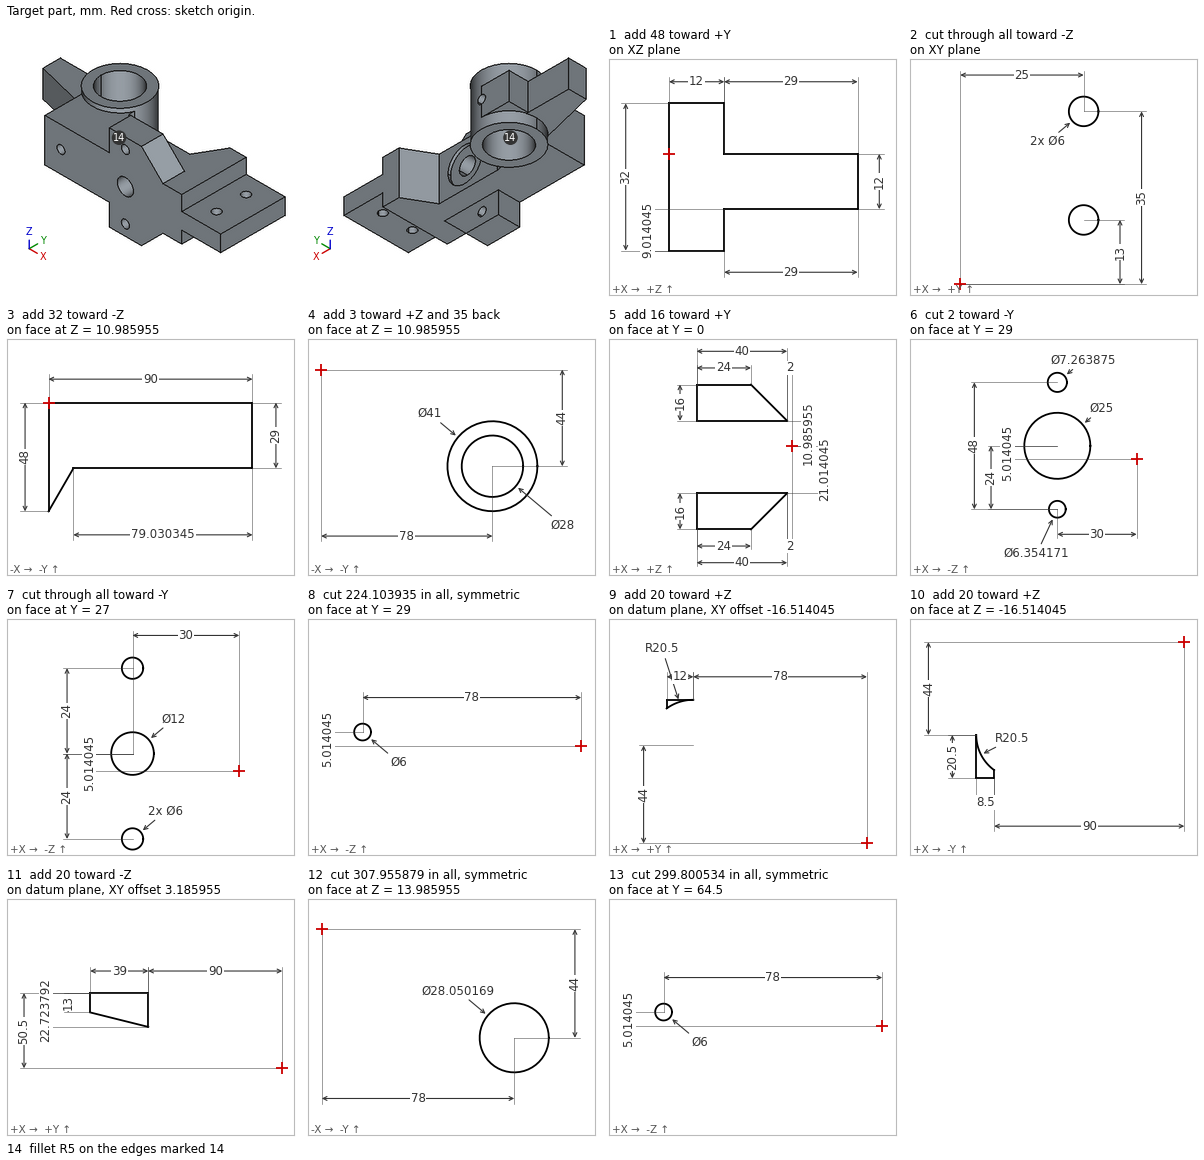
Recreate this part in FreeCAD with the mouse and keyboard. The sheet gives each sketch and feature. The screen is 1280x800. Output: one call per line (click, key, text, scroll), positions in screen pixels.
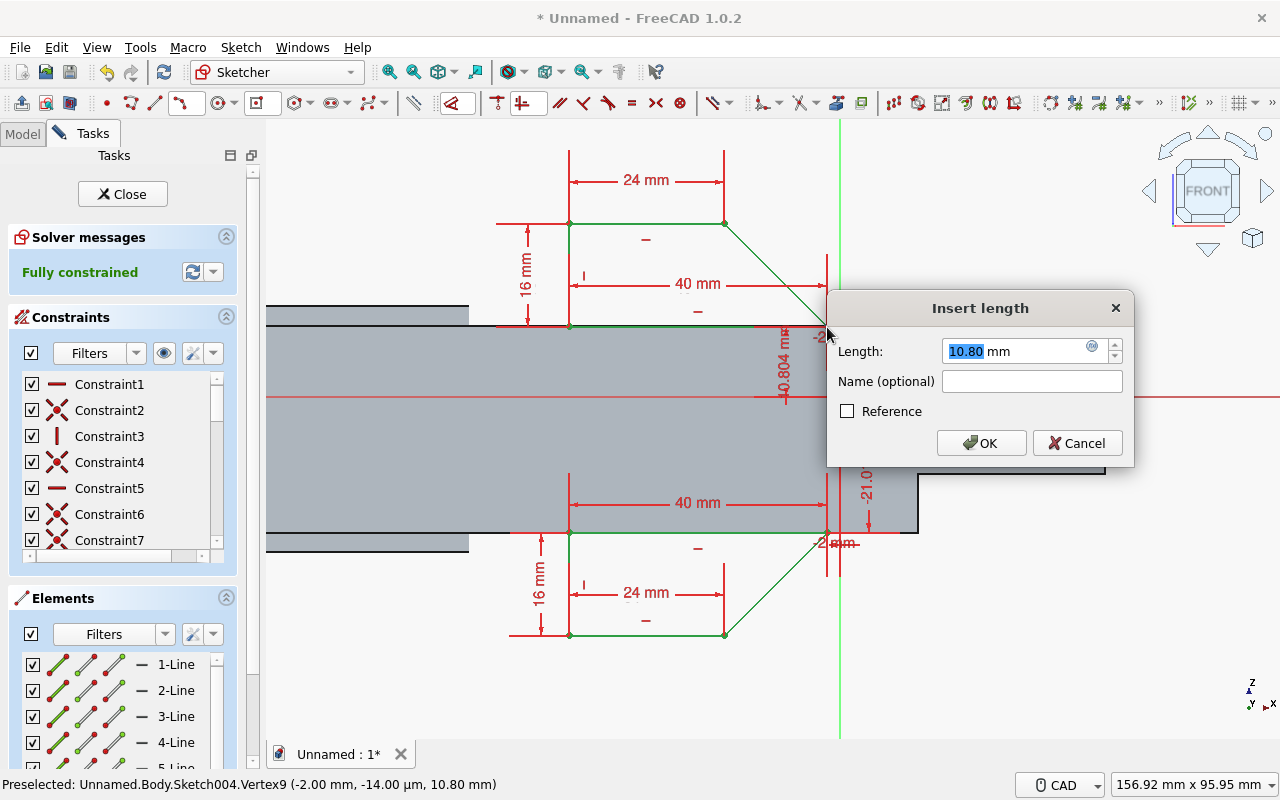
text(10.985955)
key(Return)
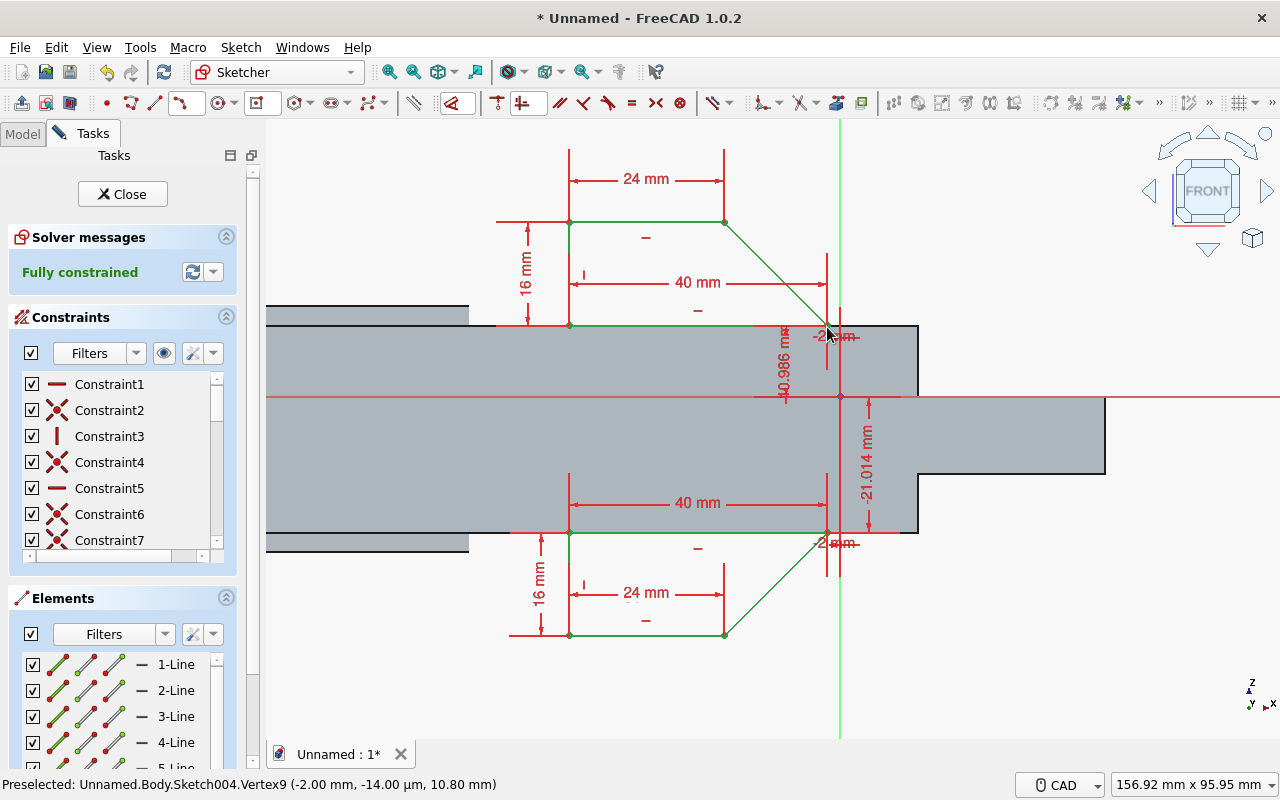
click(123, 194)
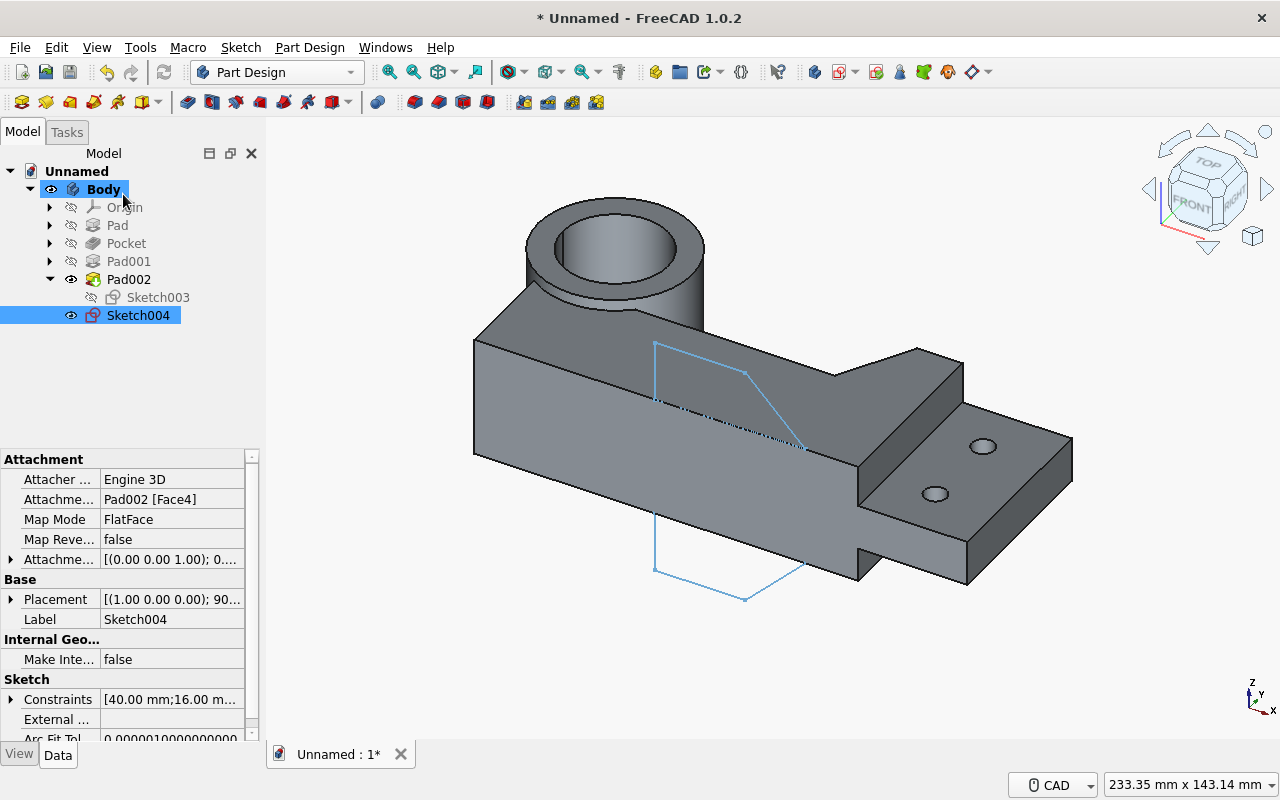
click(22, 102)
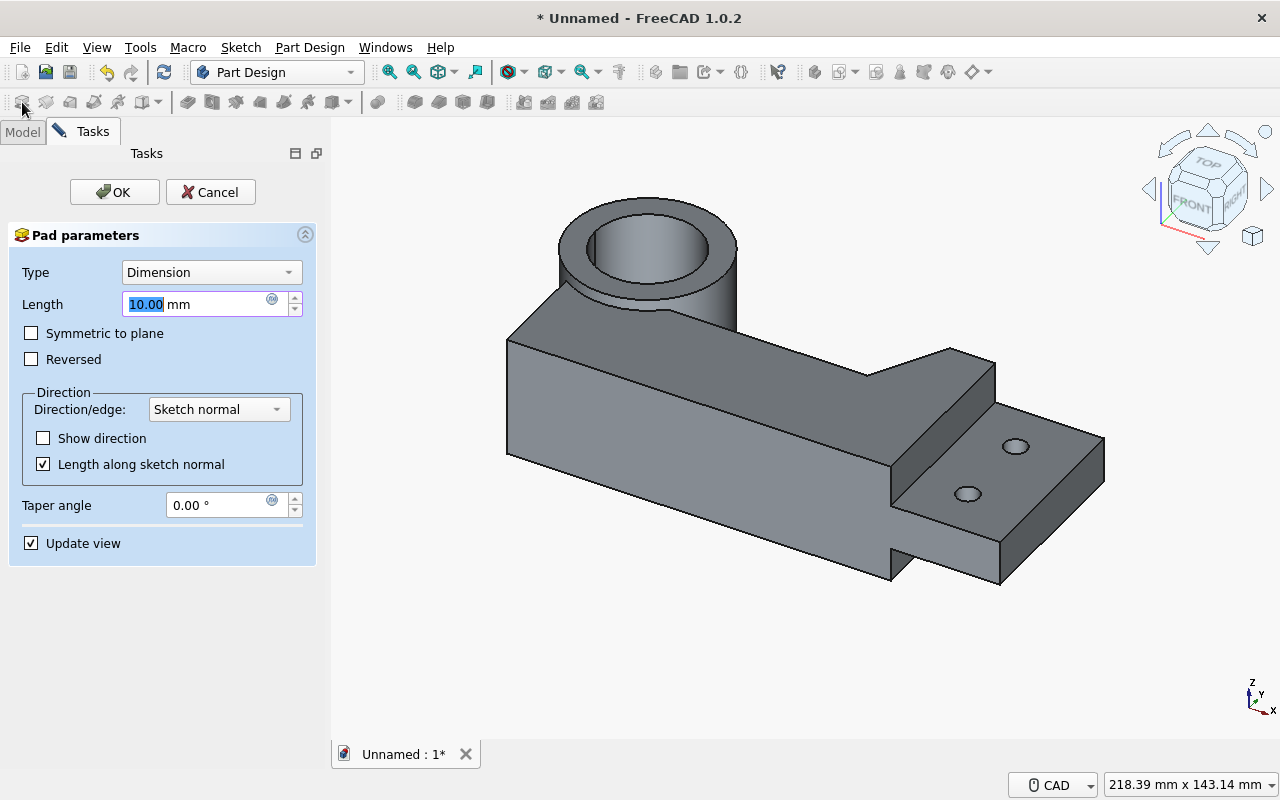
text(16)
key(Tab)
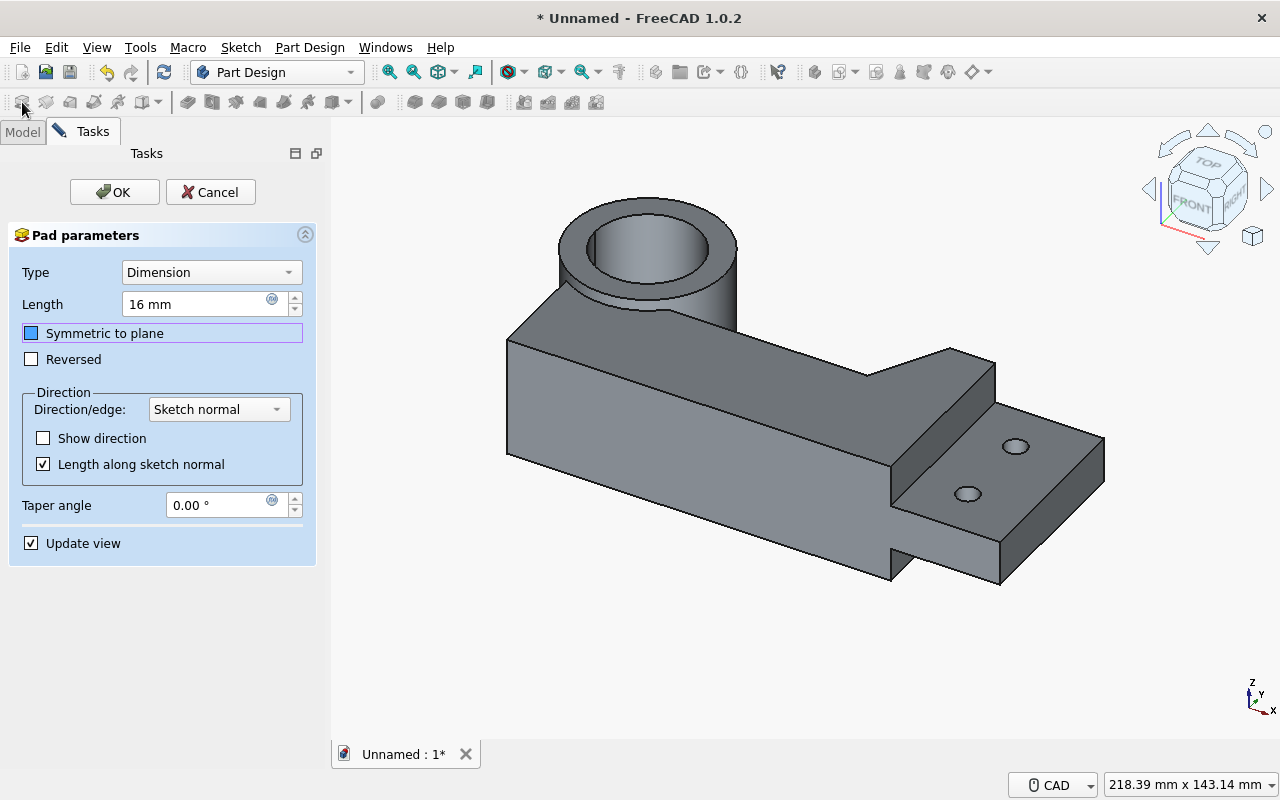
click(30, 359)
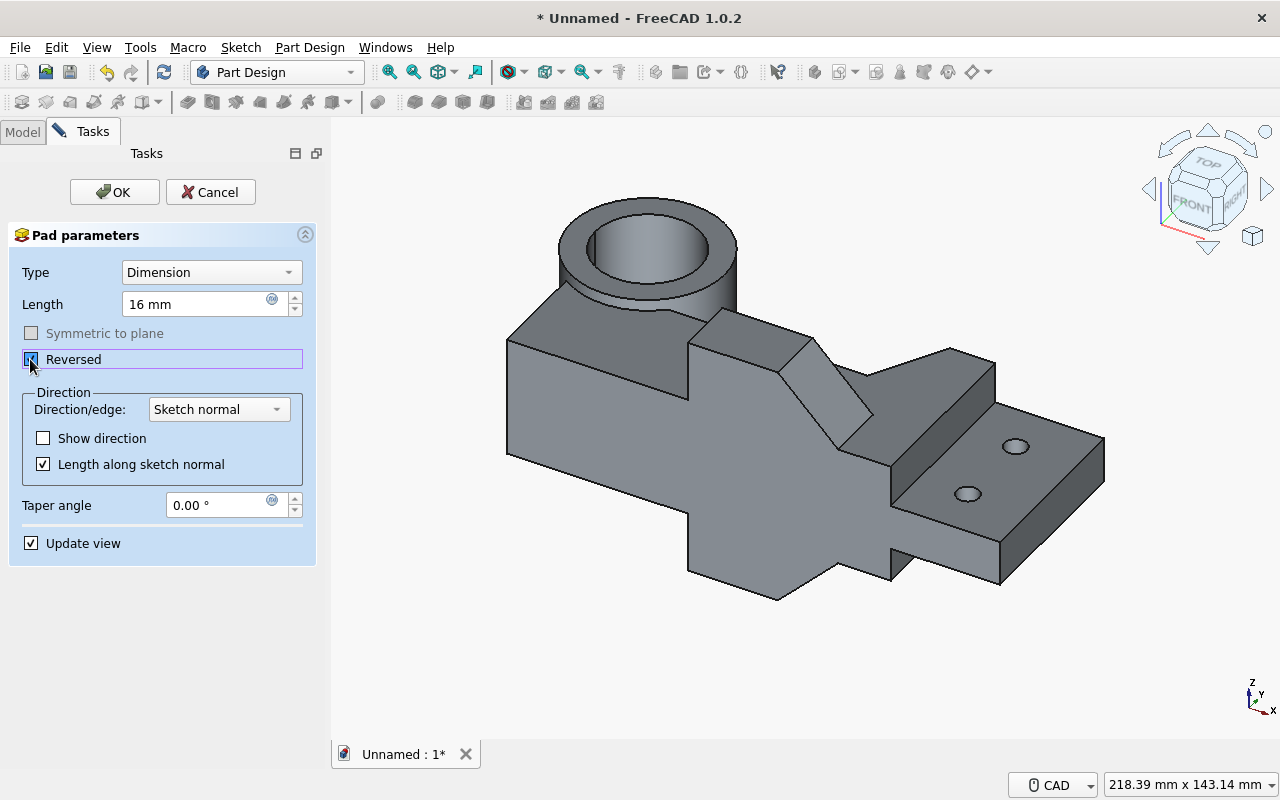
click(115, 192)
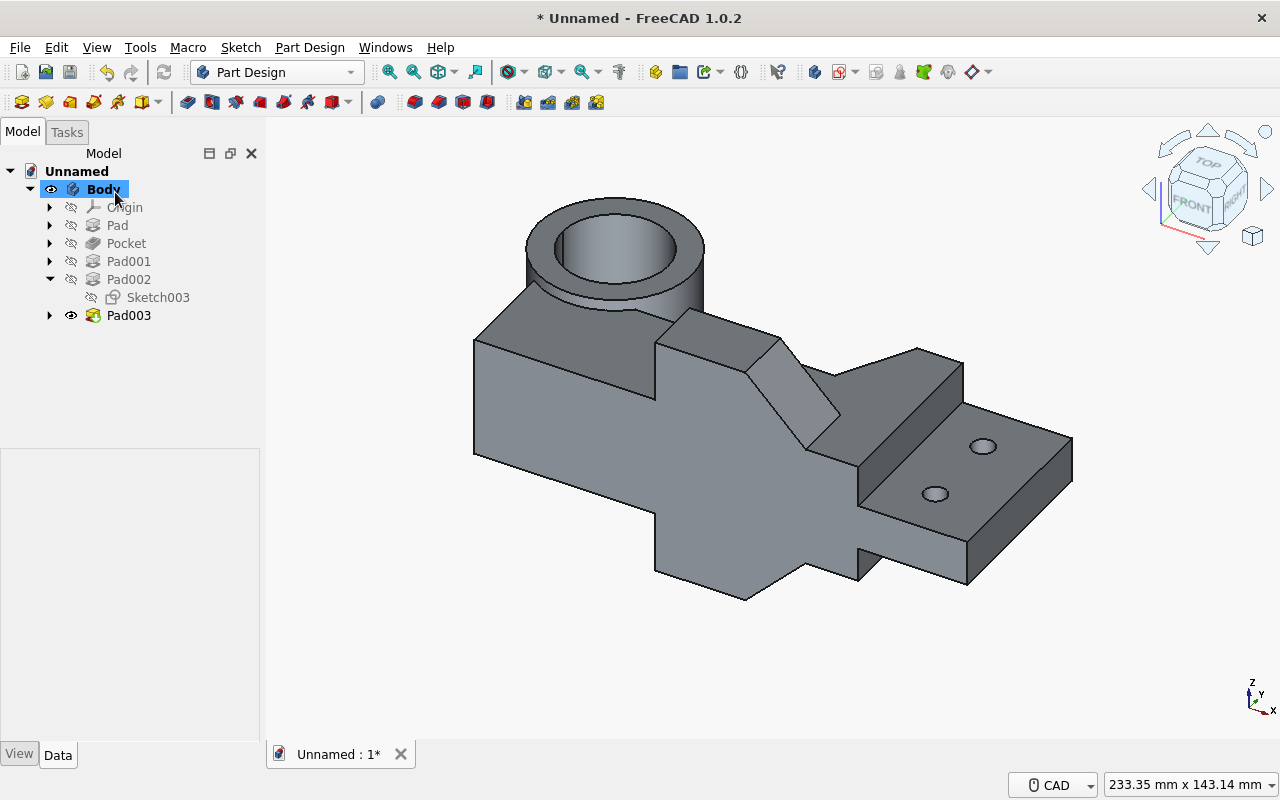
key(4)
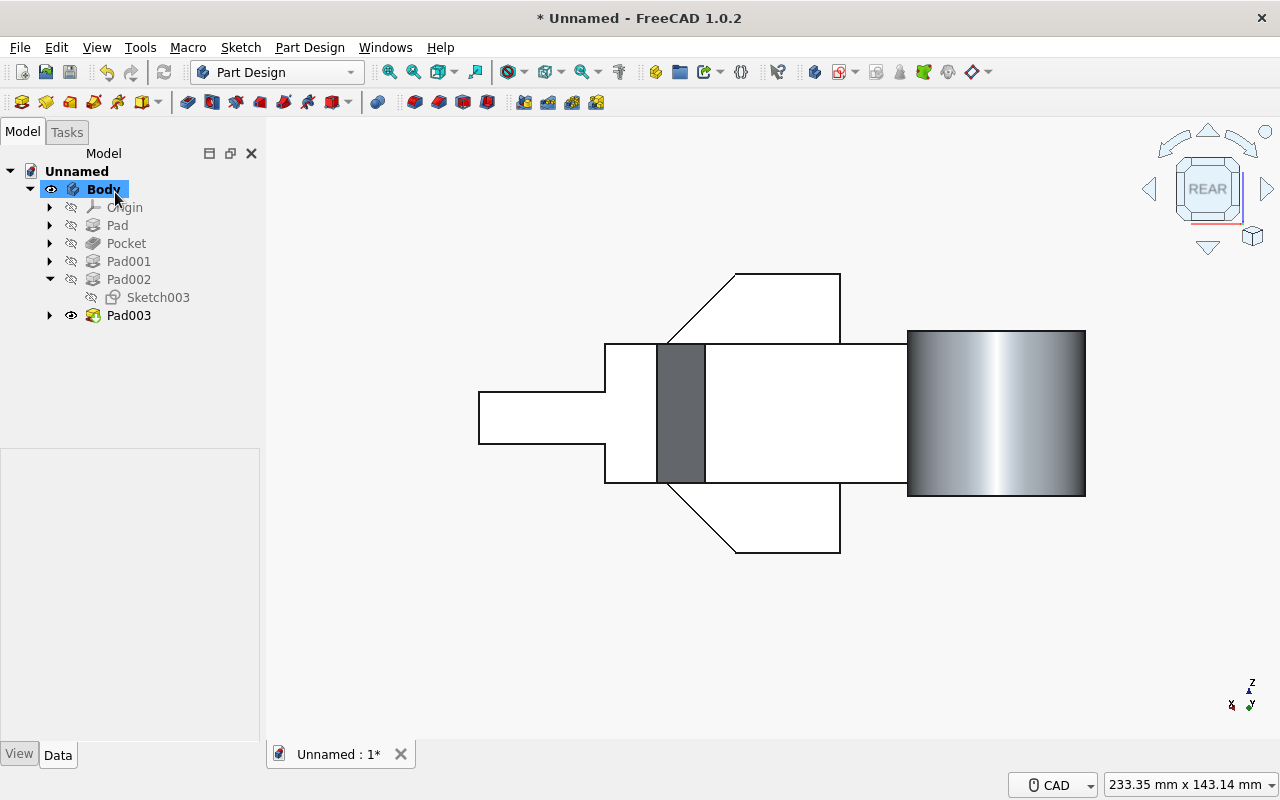
click(787, 413)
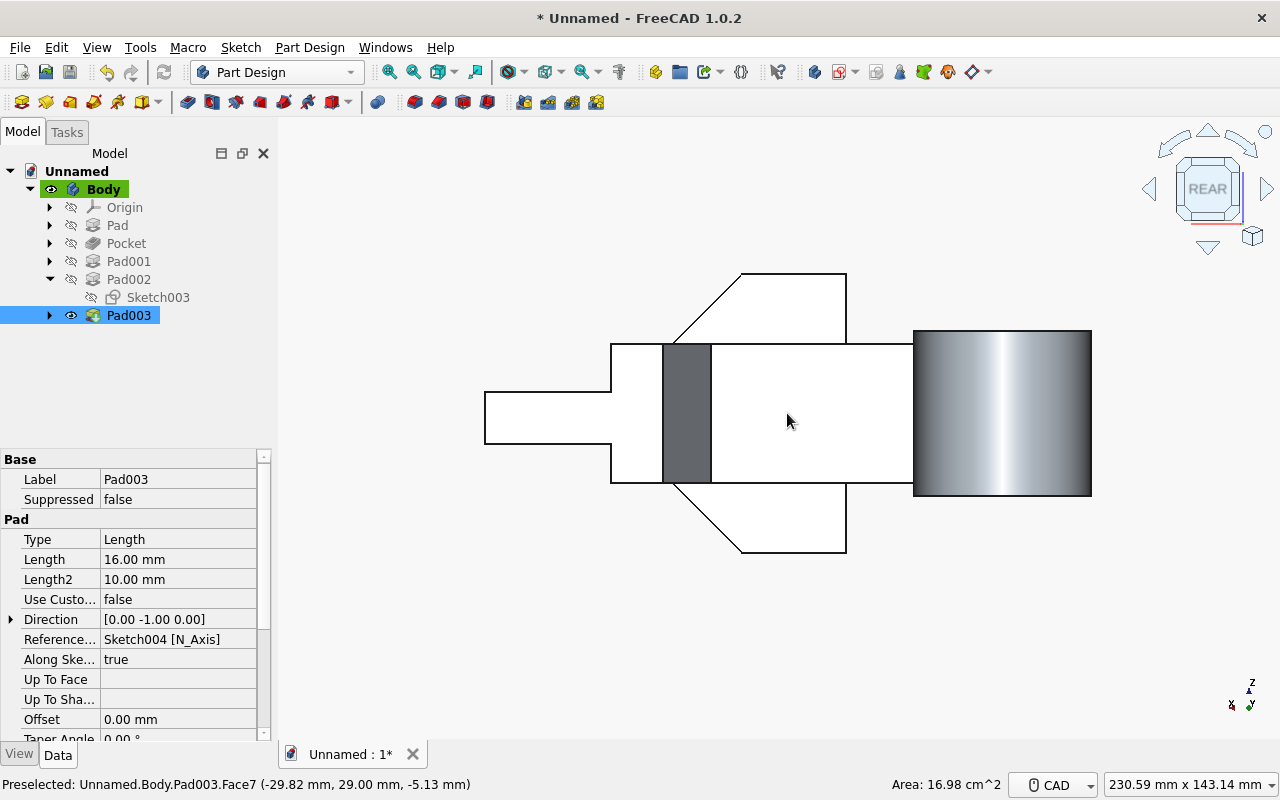
click(840, 72)